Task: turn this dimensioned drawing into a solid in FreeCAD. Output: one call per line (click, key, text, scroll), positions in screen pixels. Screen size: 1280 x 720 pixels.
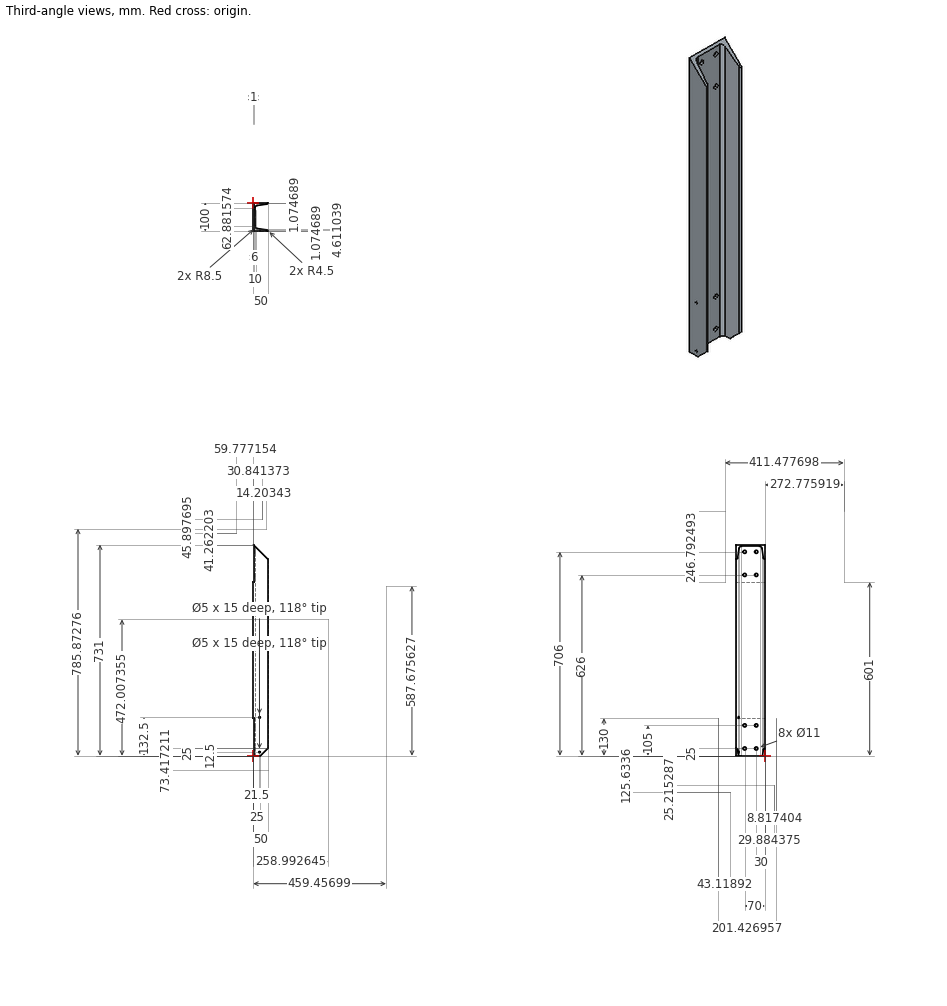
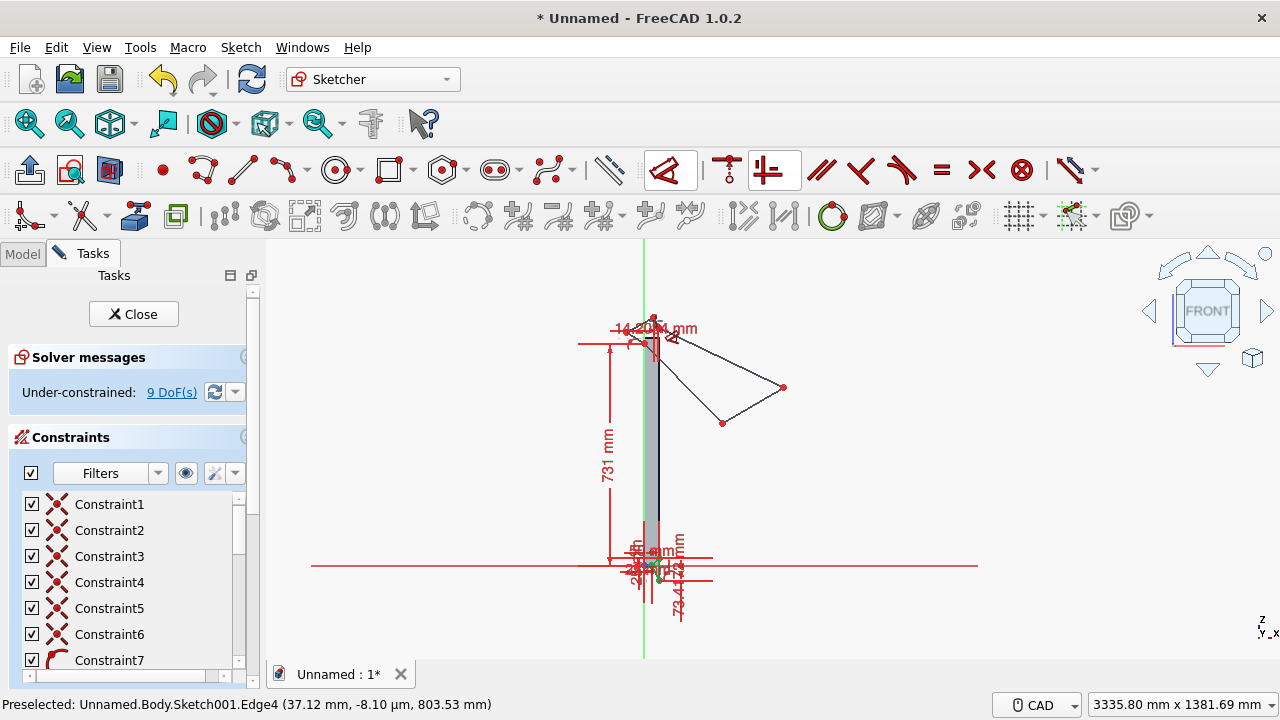
scroll(627, 332, up, 4)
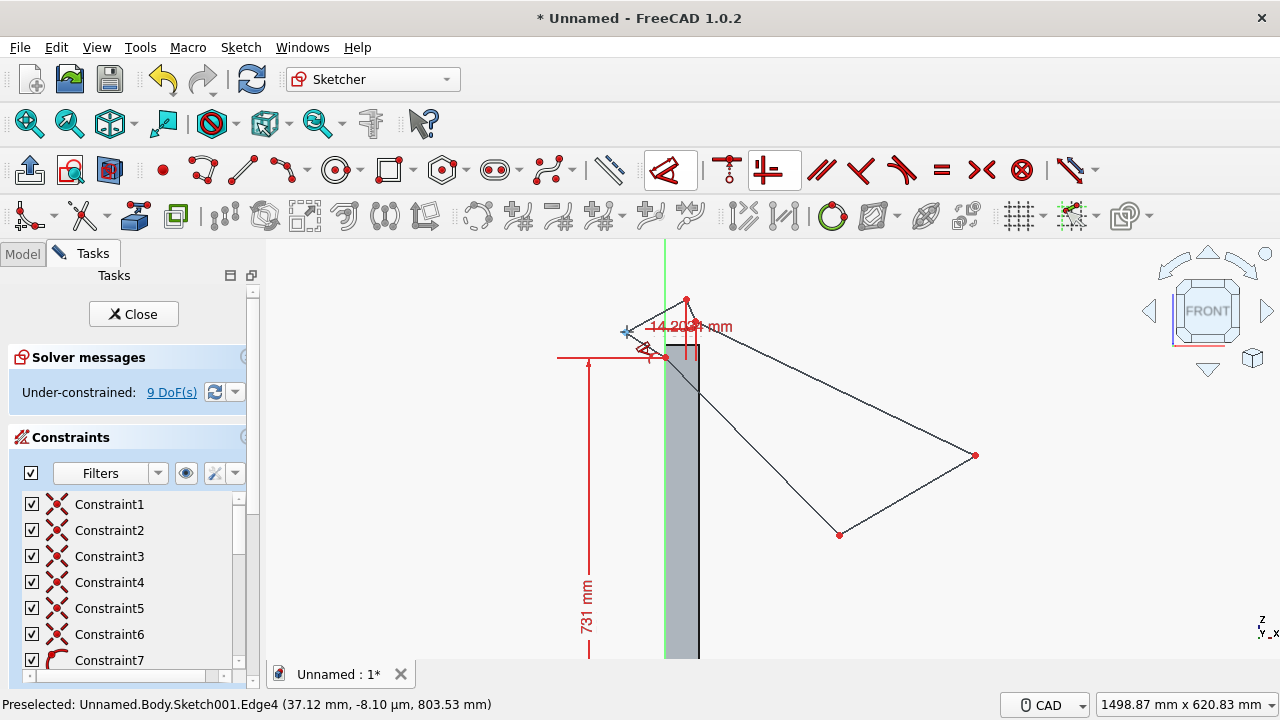
click(626, 333)
click(645, 299)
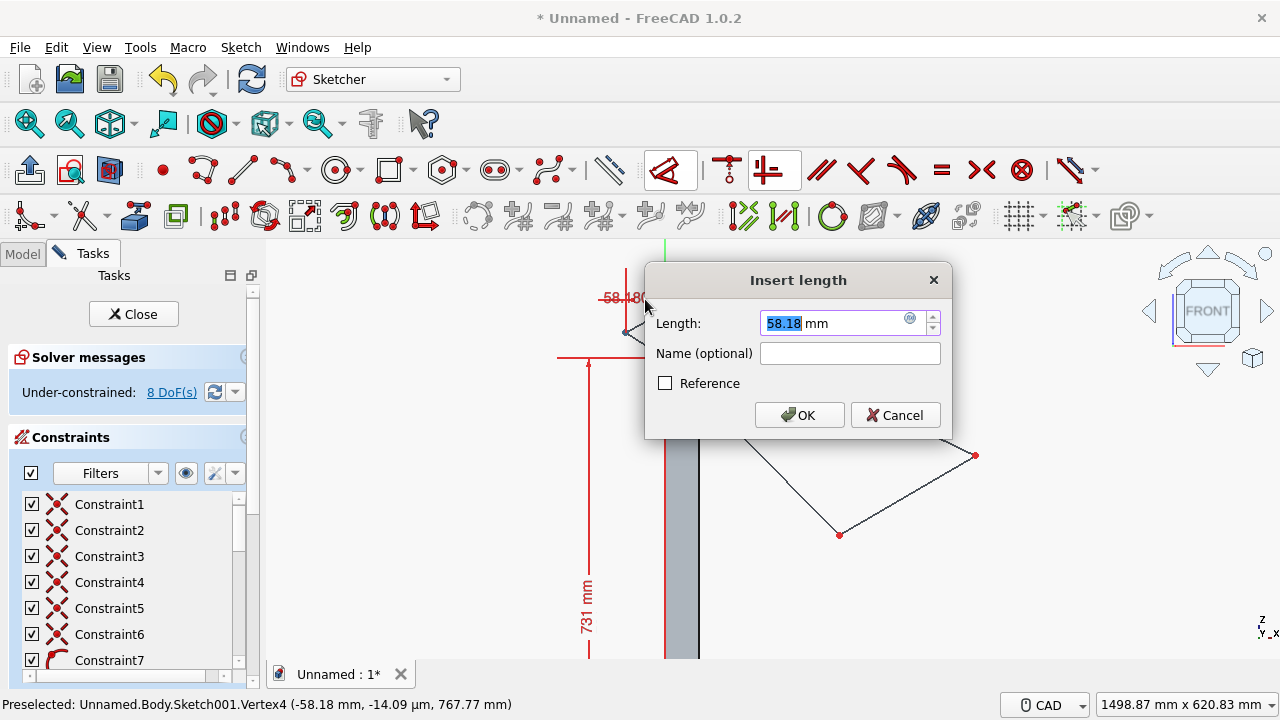
text(59.777154)
key(Return)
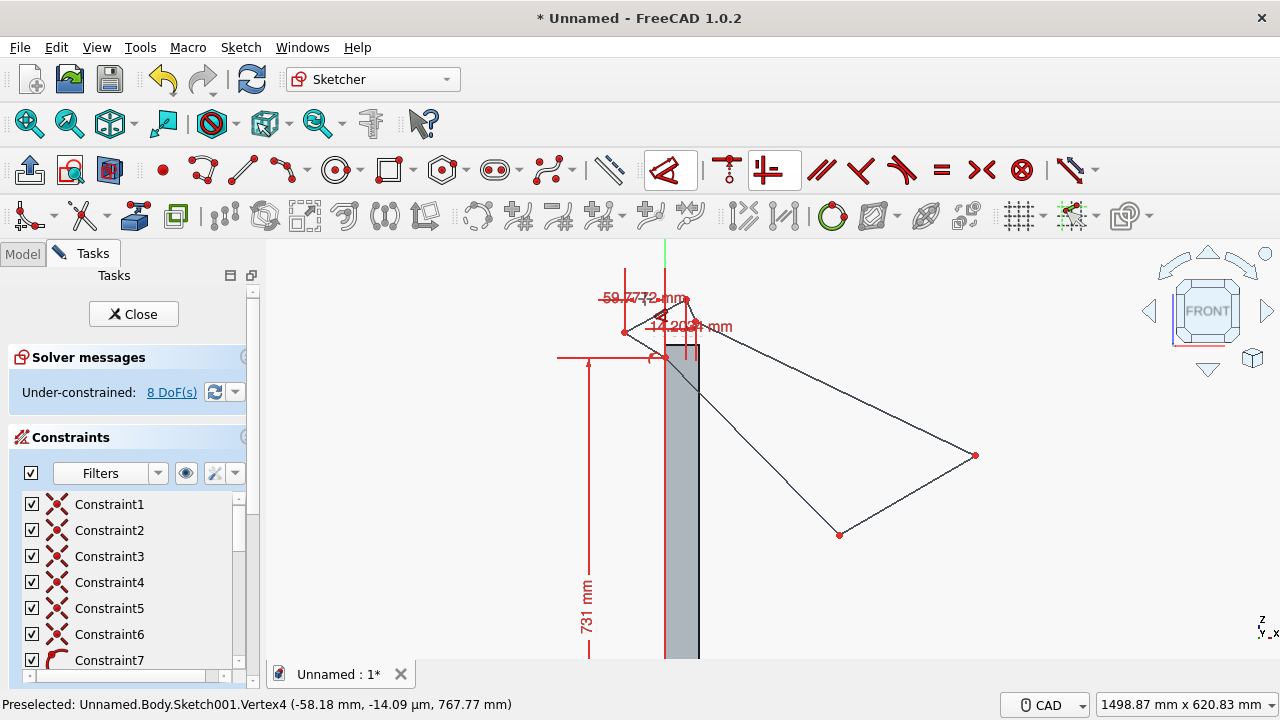
scroll(686, 300, up, 4)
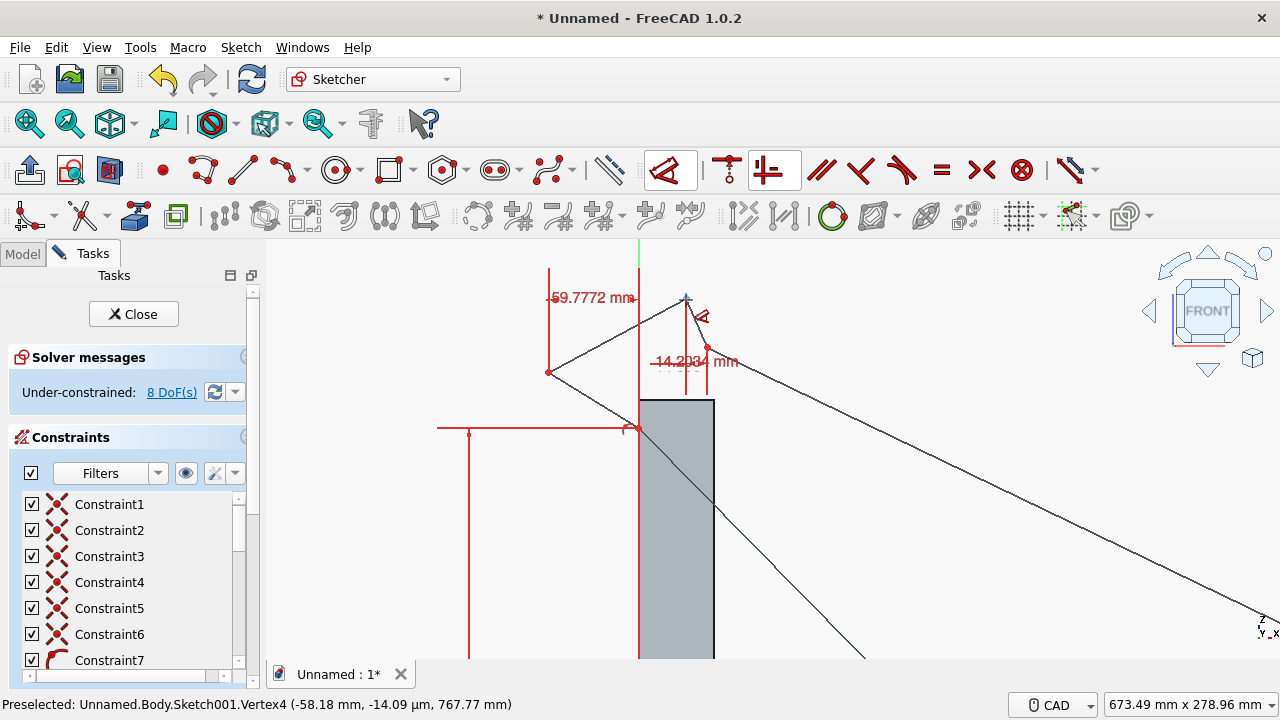
click(686, 299)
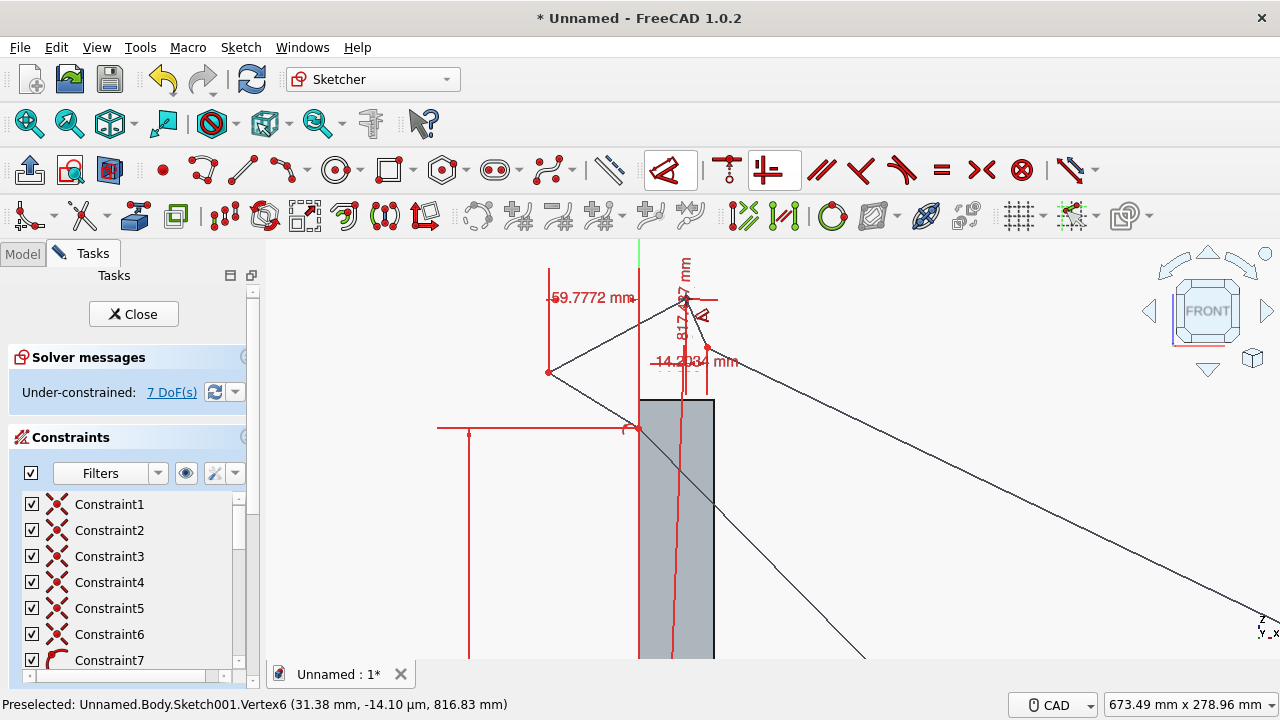
key(Escape)
key(Escape)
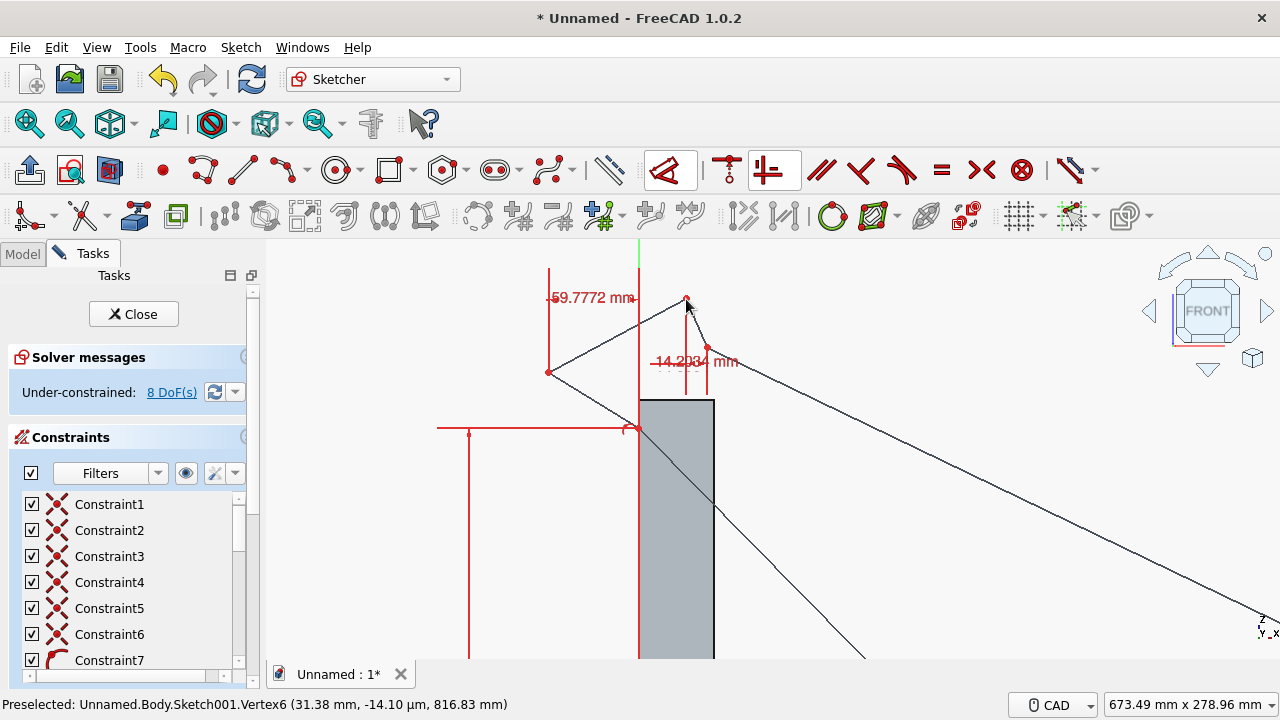
click(686, 299)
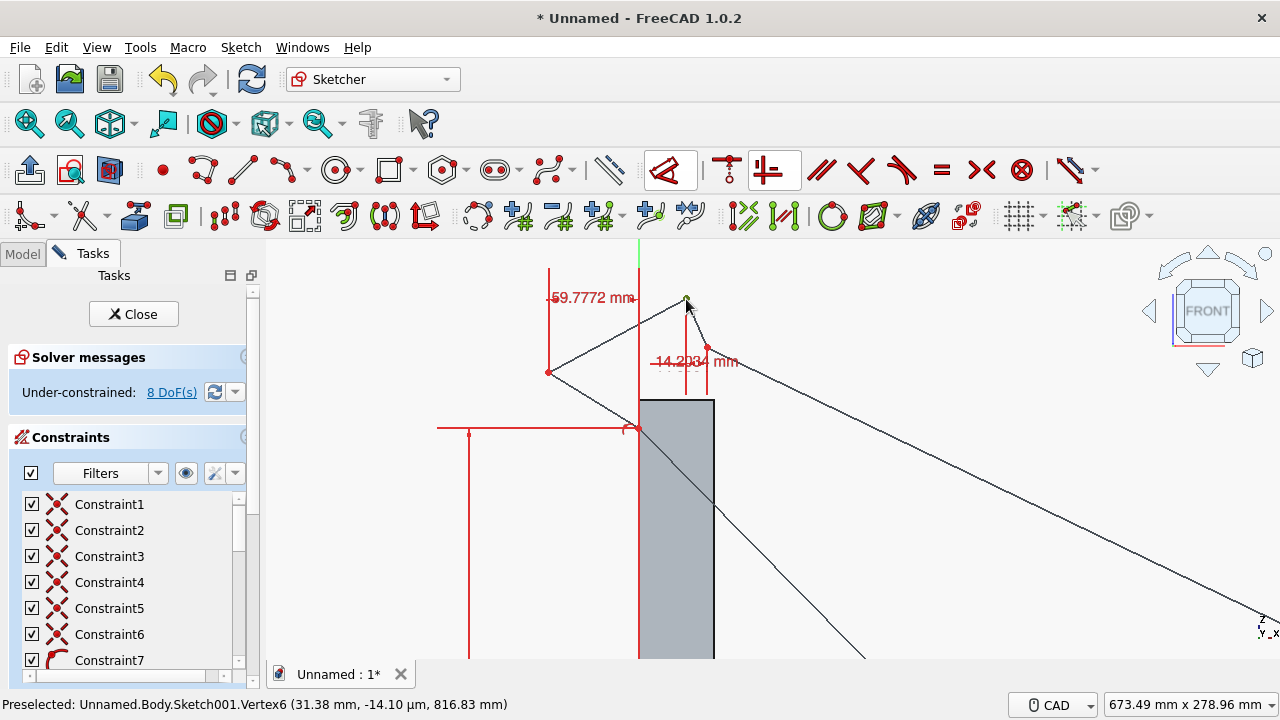
key(l)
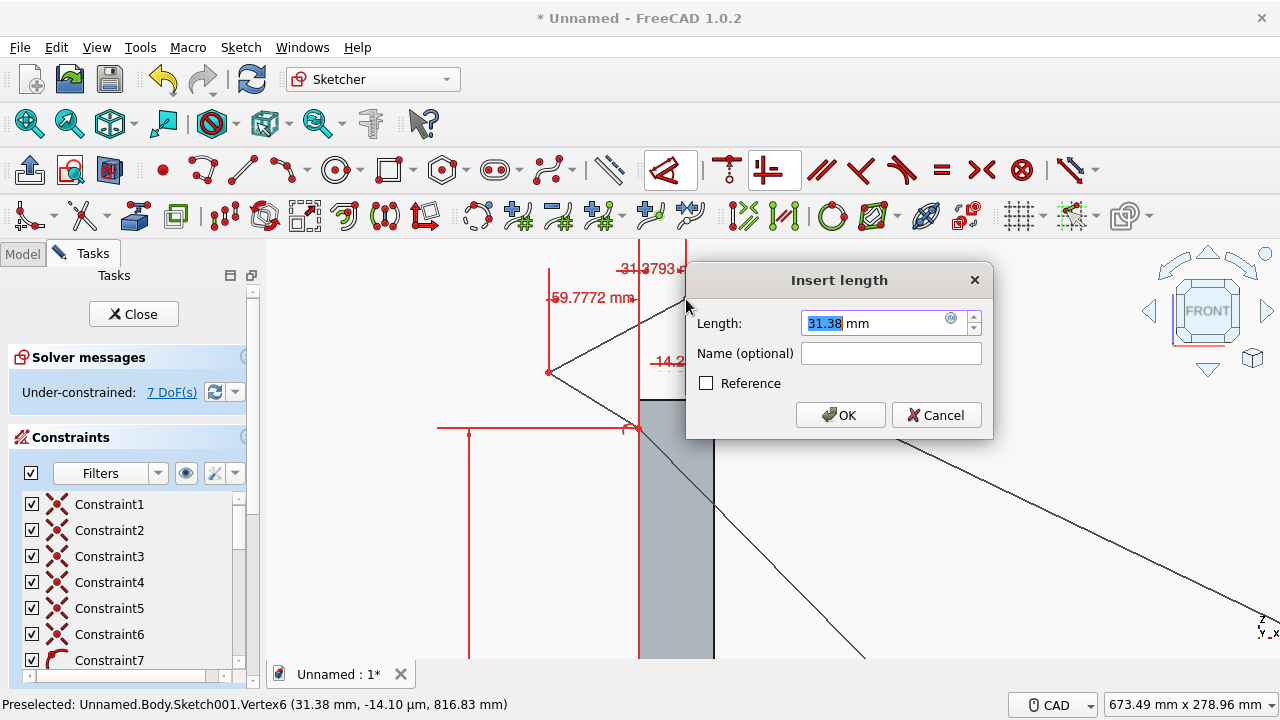
text(30.841373)
key(Return)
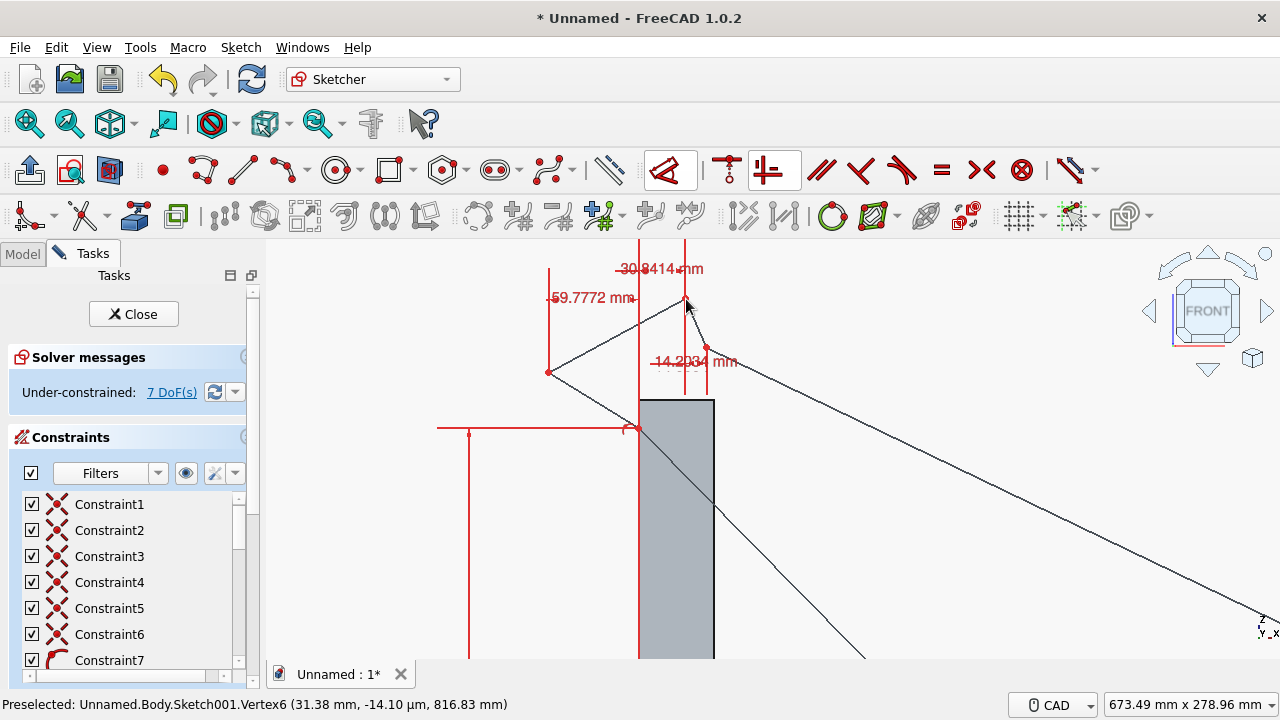
scroll(645, 322, down, 8)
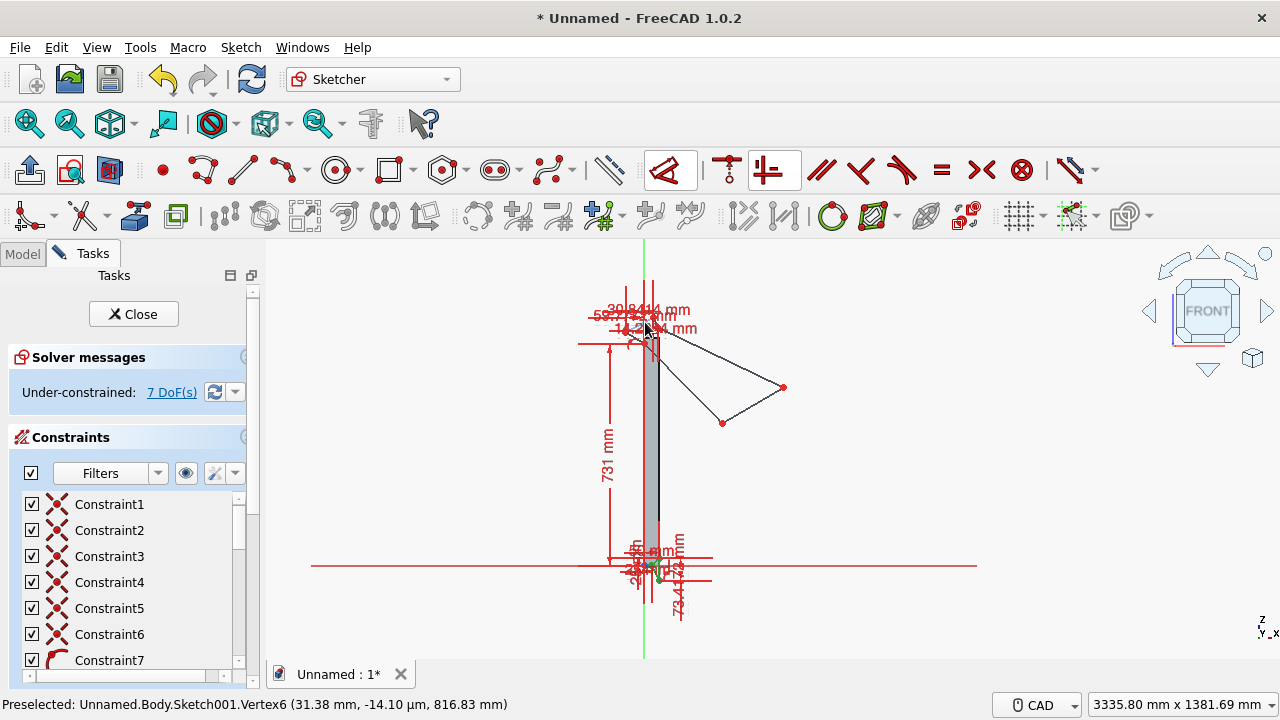
click(658, 327)